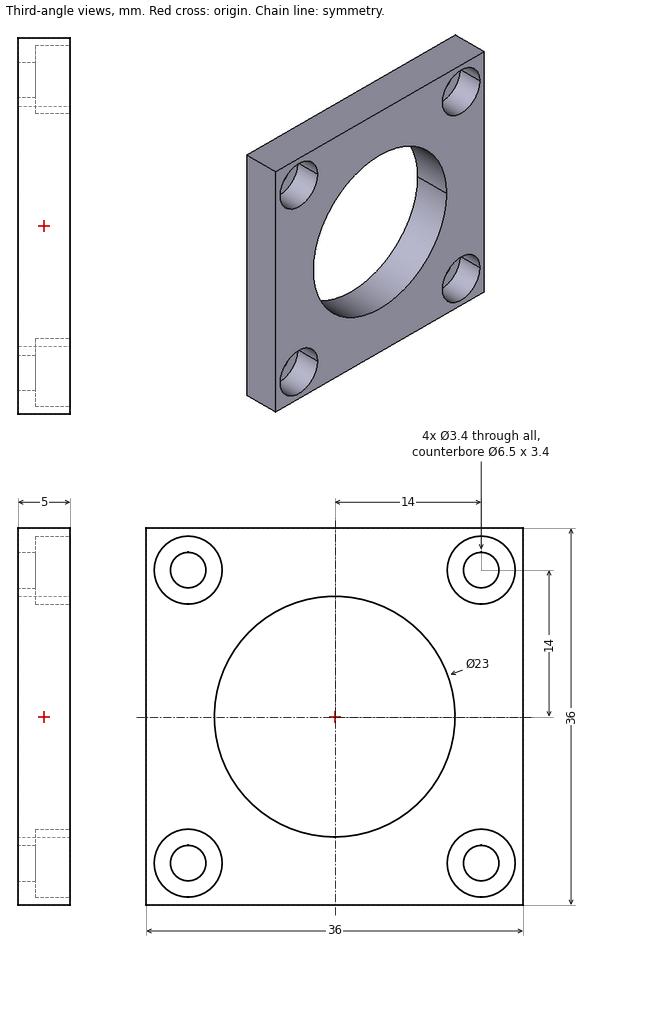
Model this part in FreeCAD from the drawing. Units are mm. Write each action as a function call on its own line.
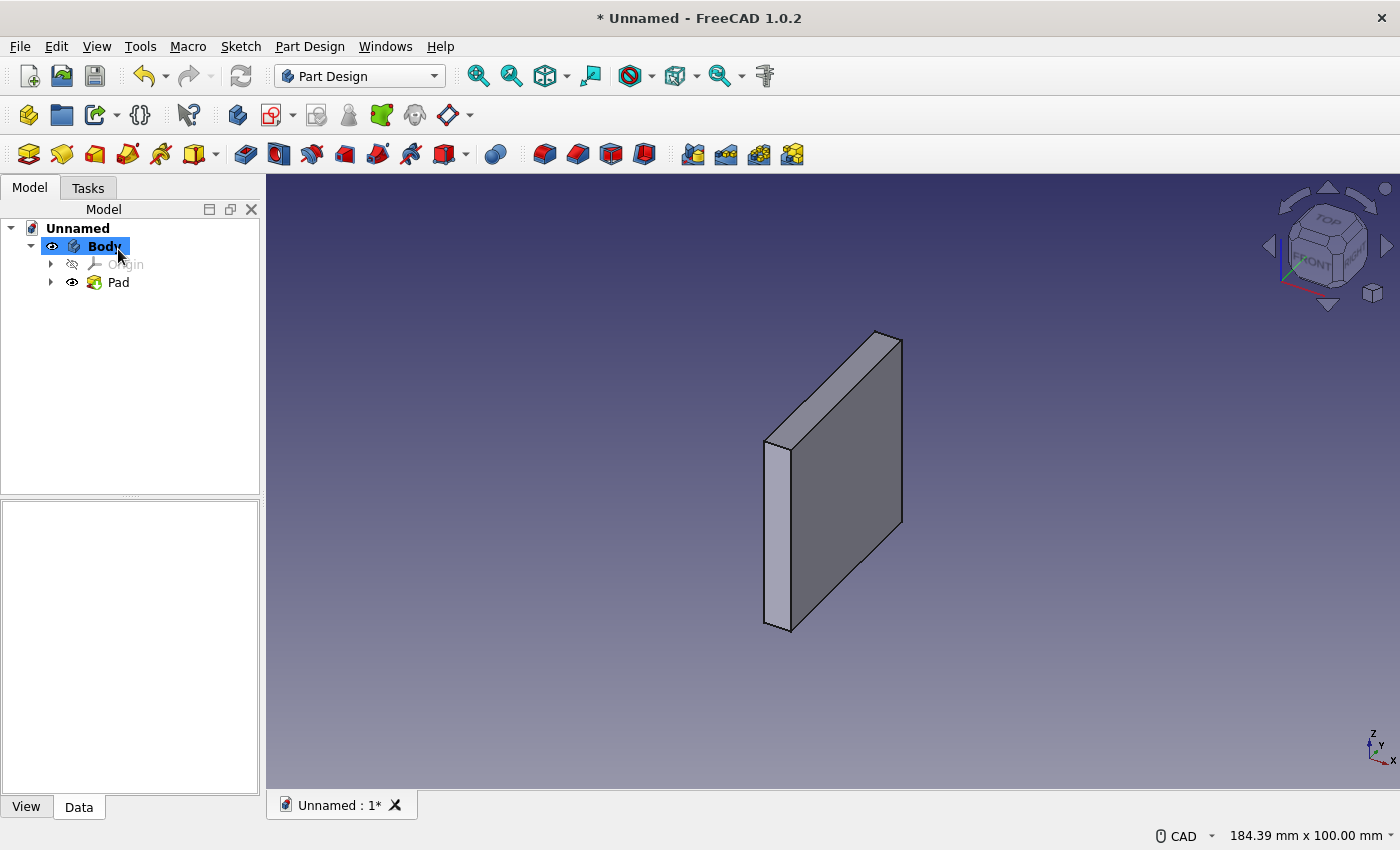
click(846, 485)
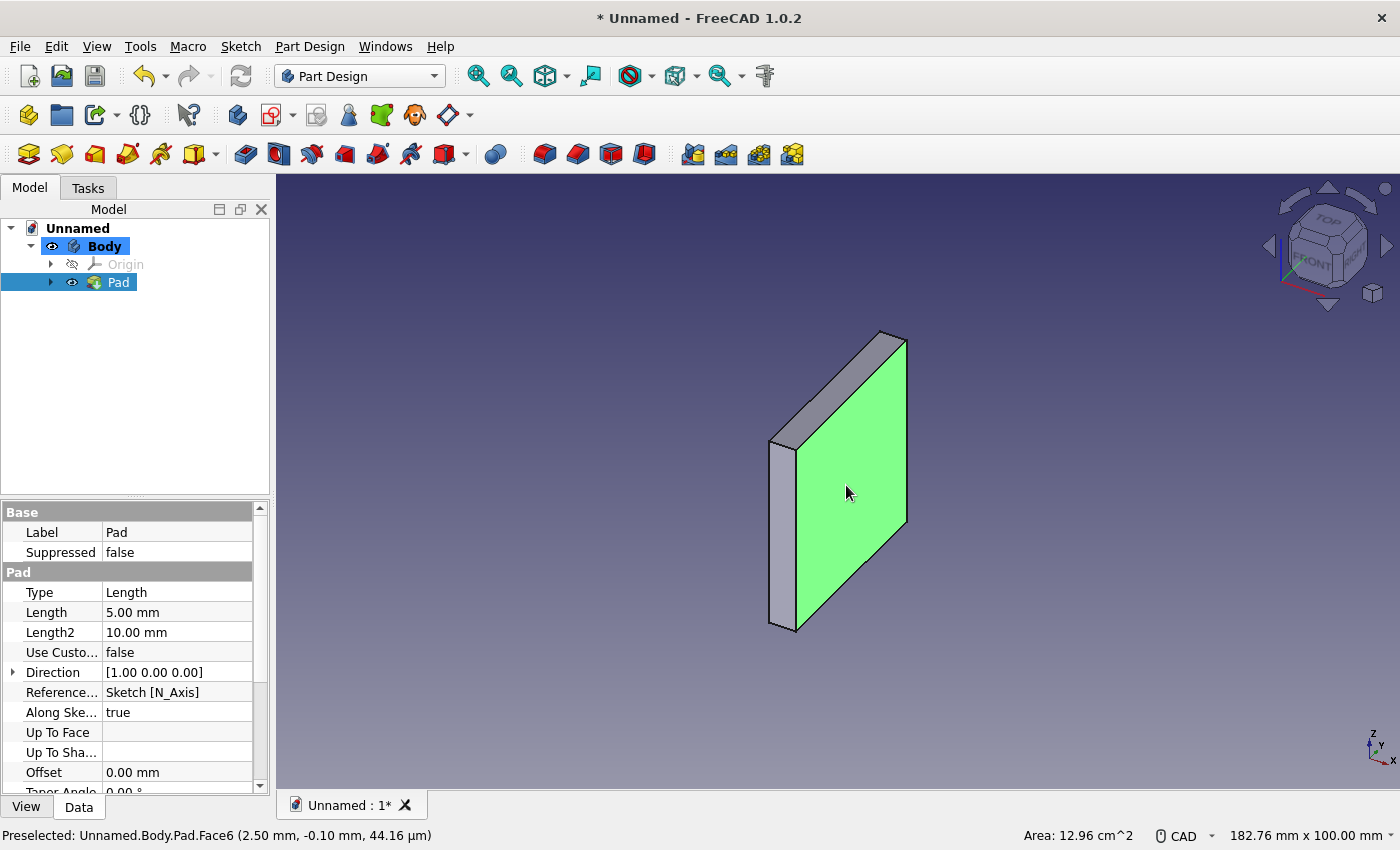
click(270, 116)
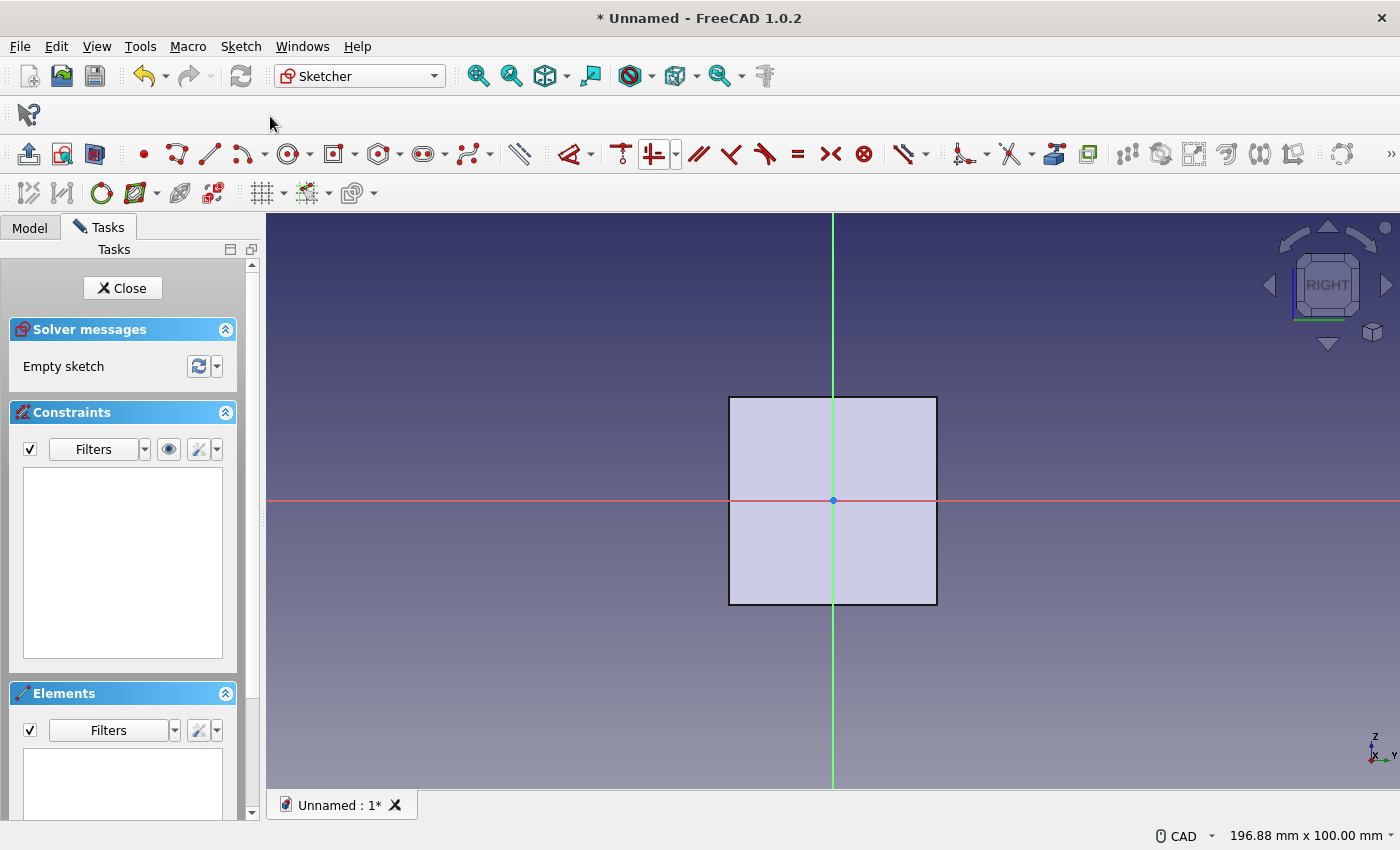
scroll(889, 501, up, 4)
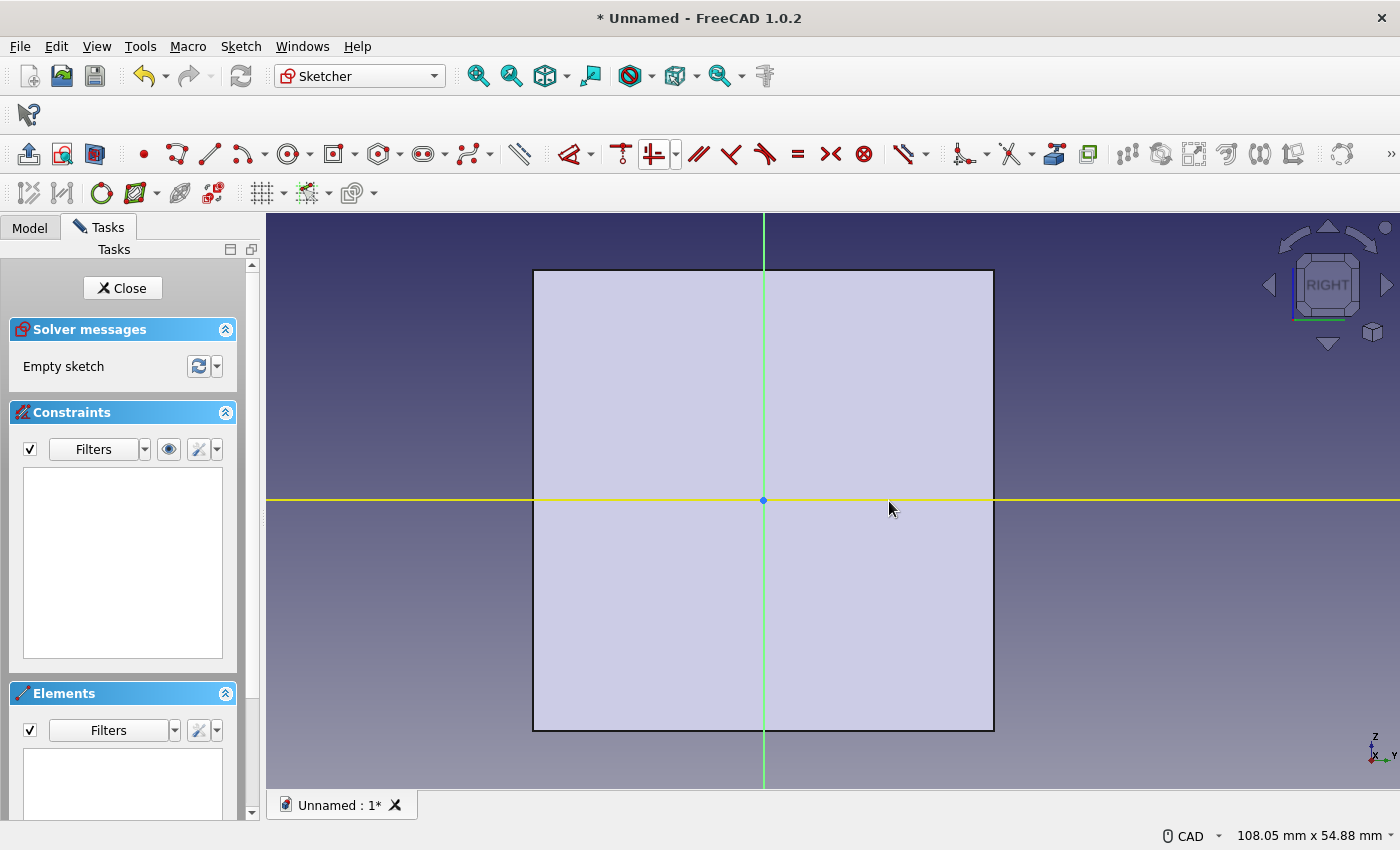
click(288, 154)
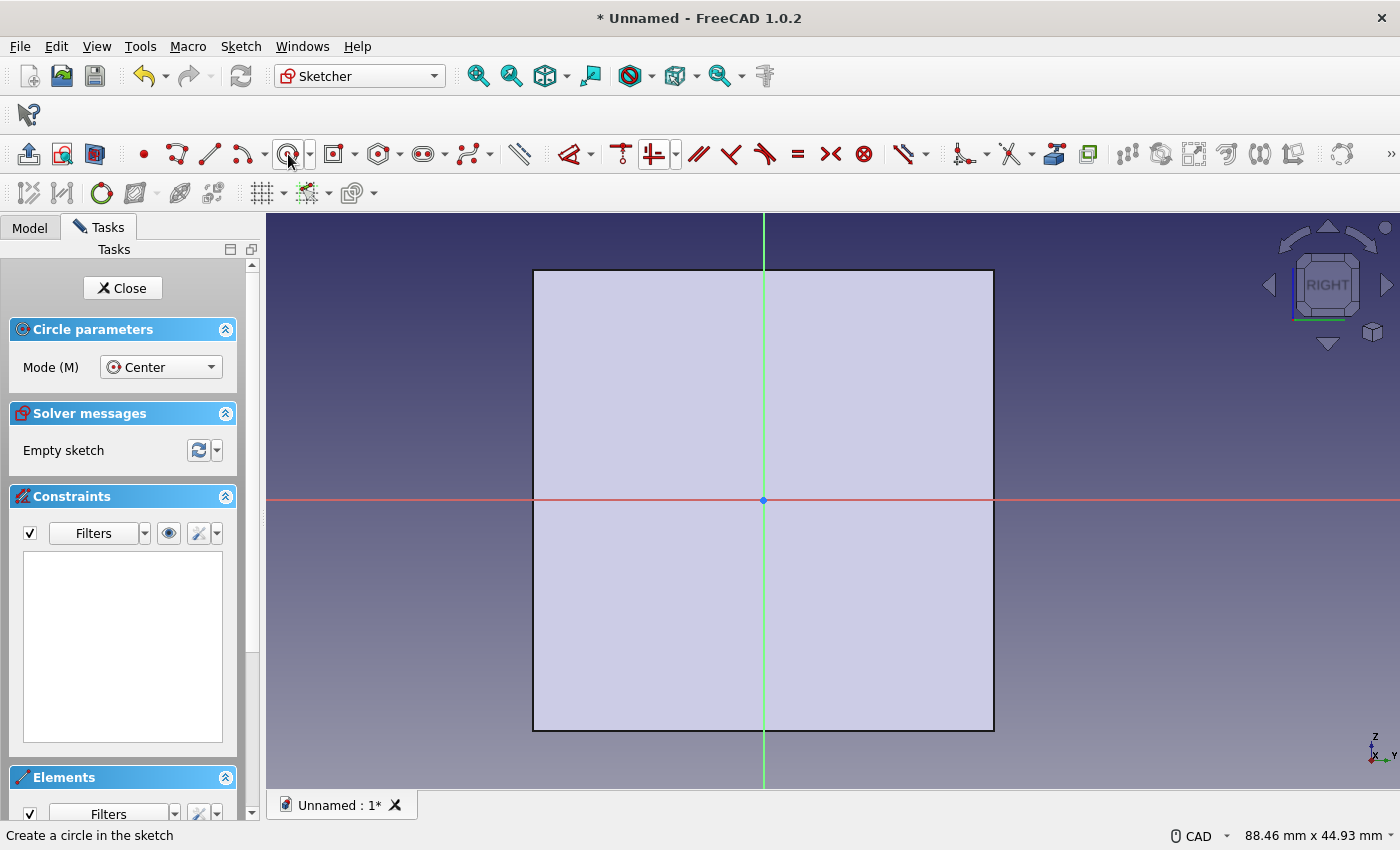
click(943, 321)
click(959, 306)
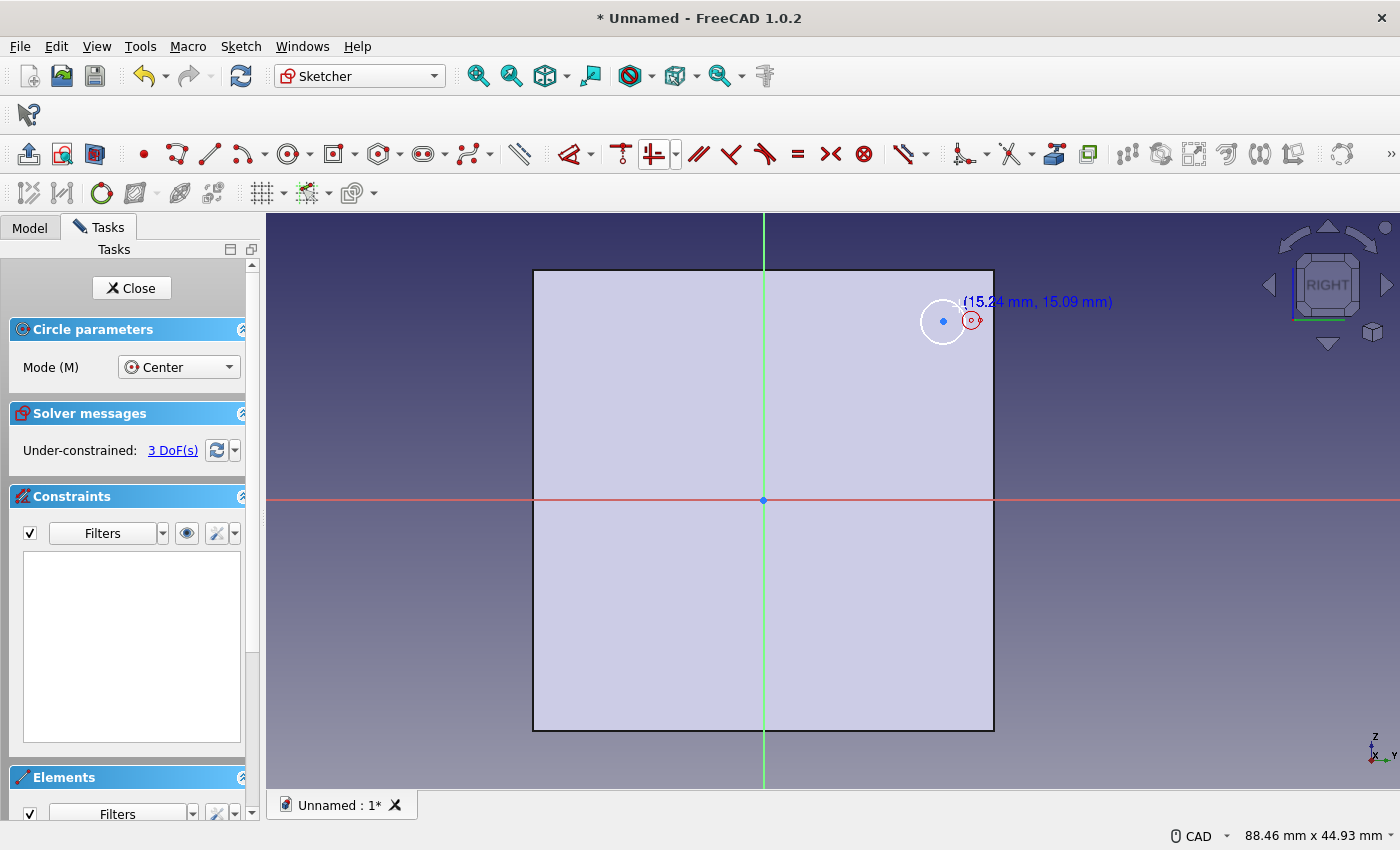
click(943, 680)
click(959, 664)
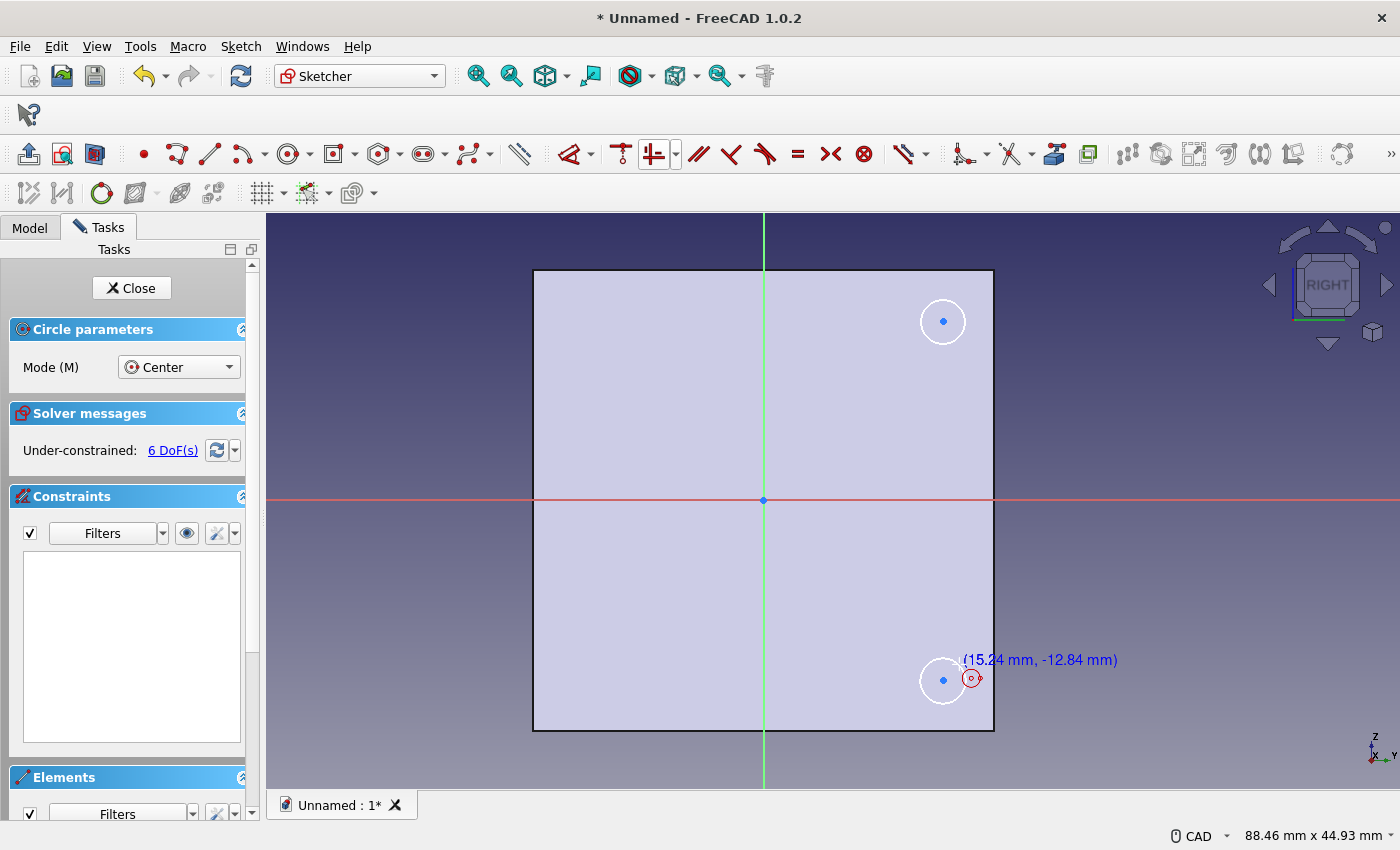
click(584, 321)
click(600, 306)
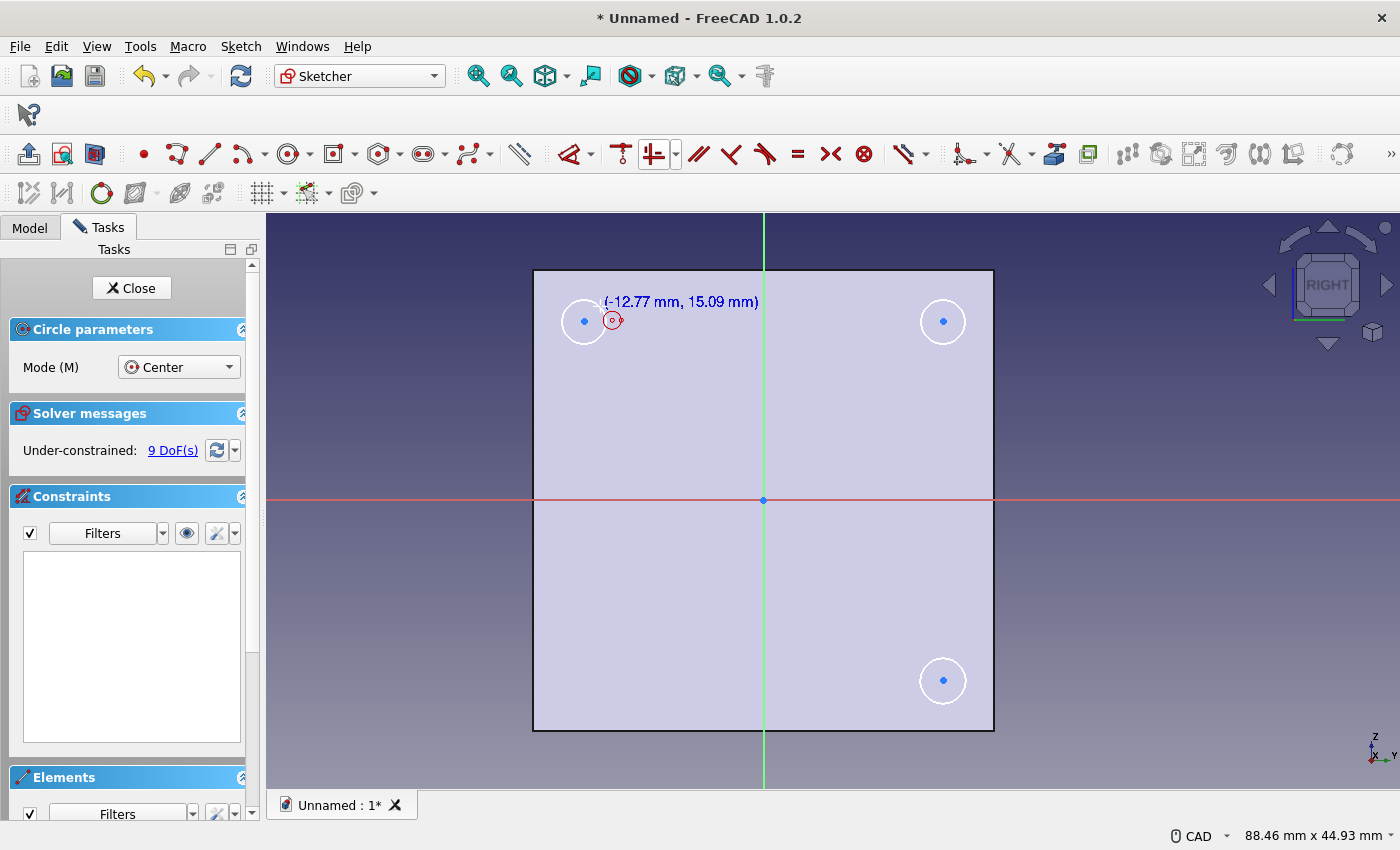
click(584, 680)
click(600, 664)
key(Escape)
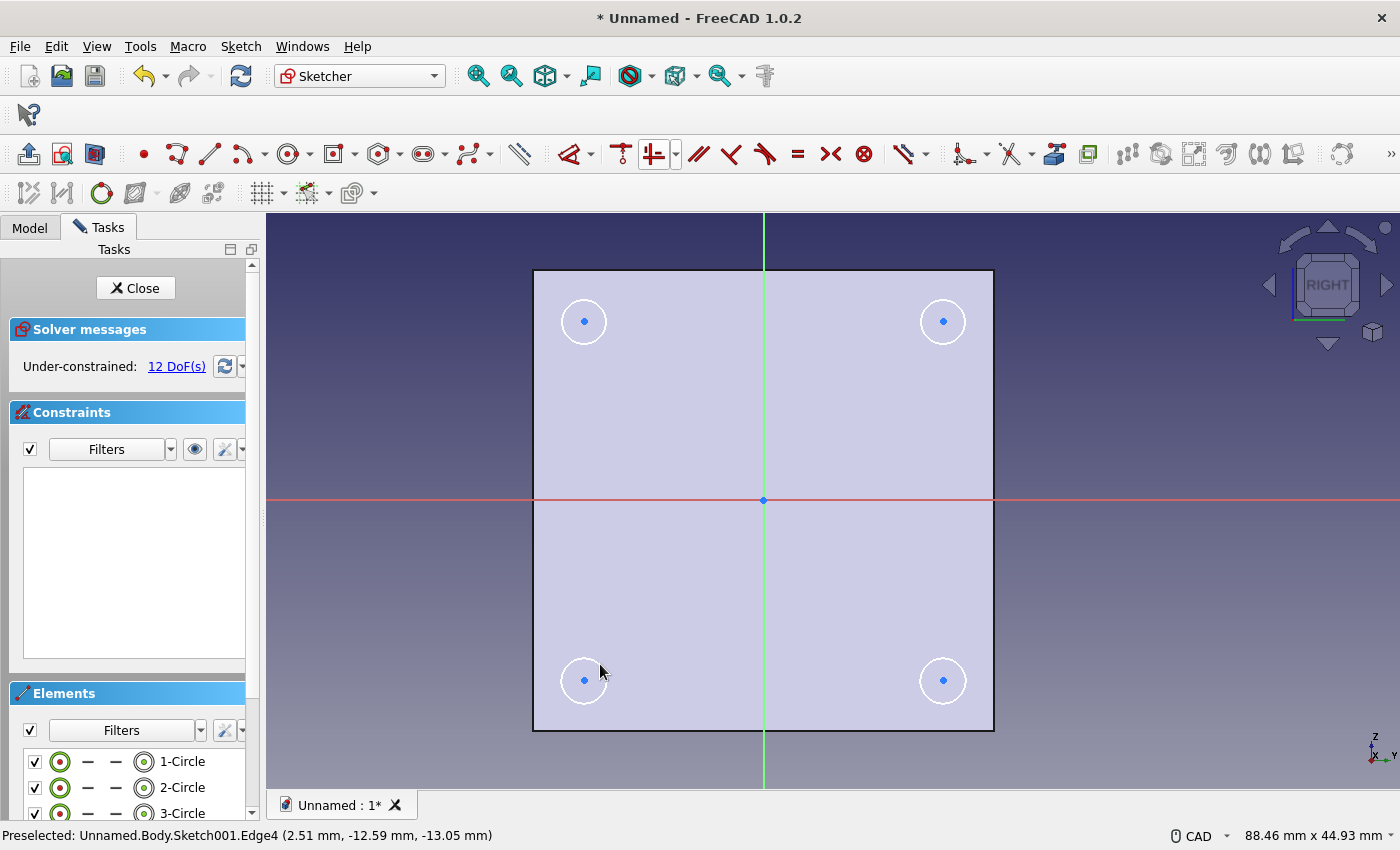
click(958, 306)